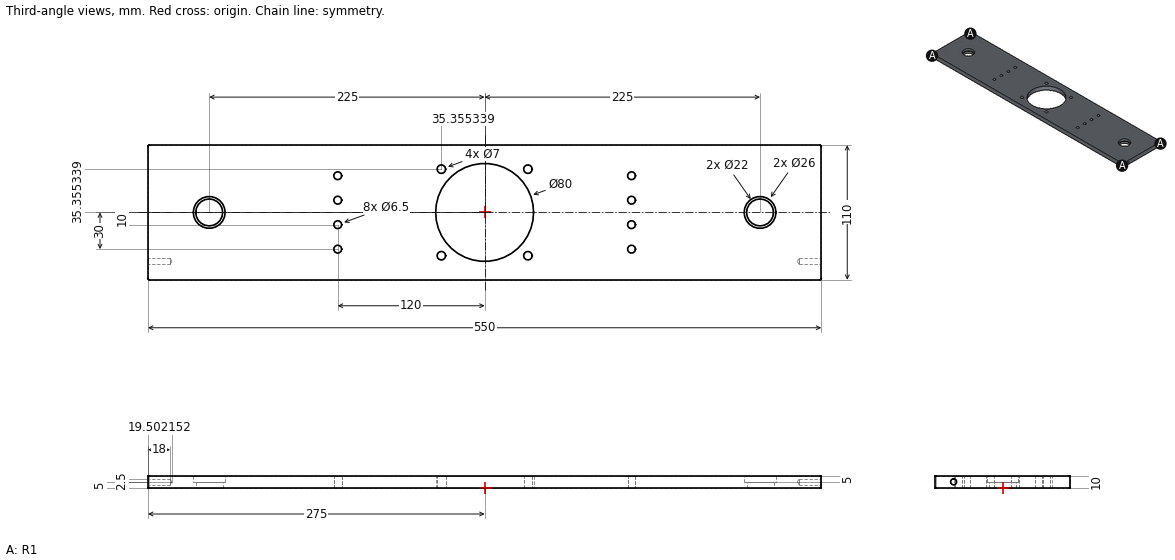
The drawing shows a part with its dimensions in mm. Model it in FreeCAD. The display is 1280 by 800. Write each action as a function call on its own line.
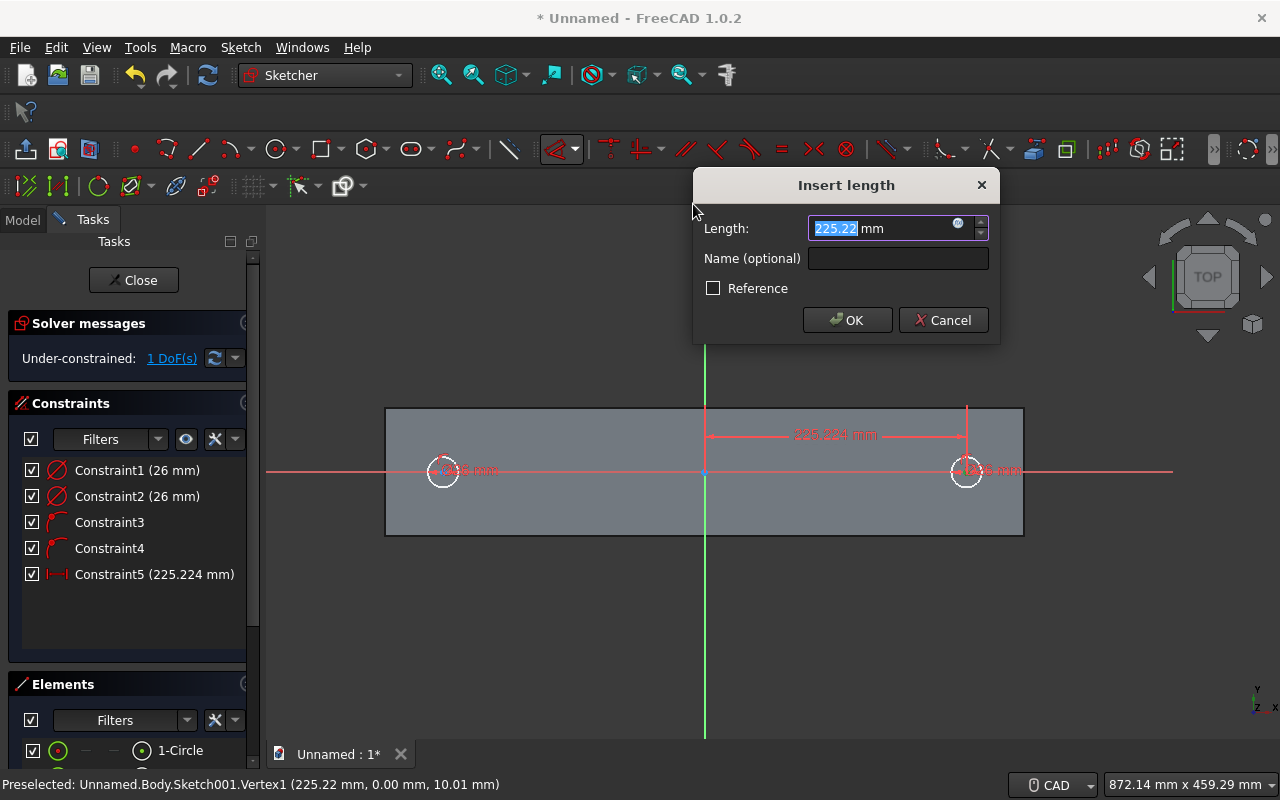
text(225)
key(Return)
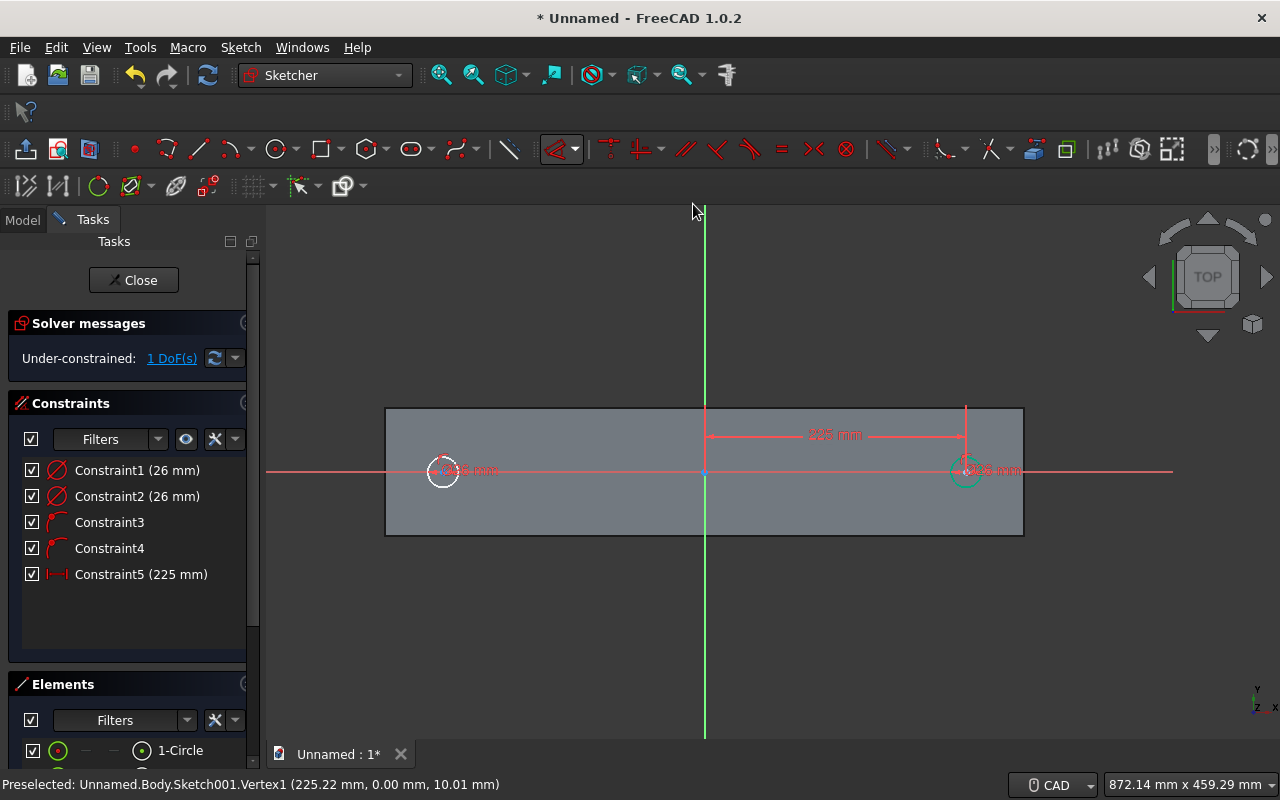
click(443, 472)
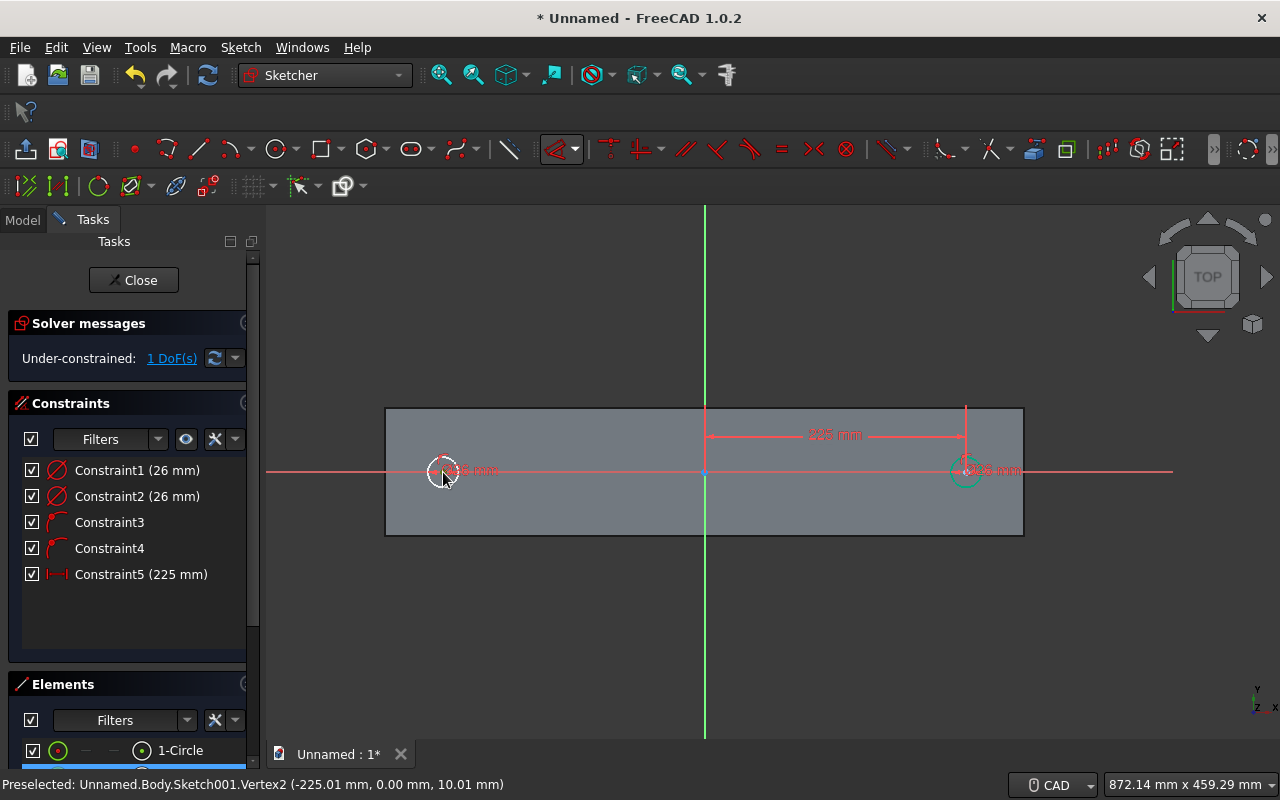
click(578, 150)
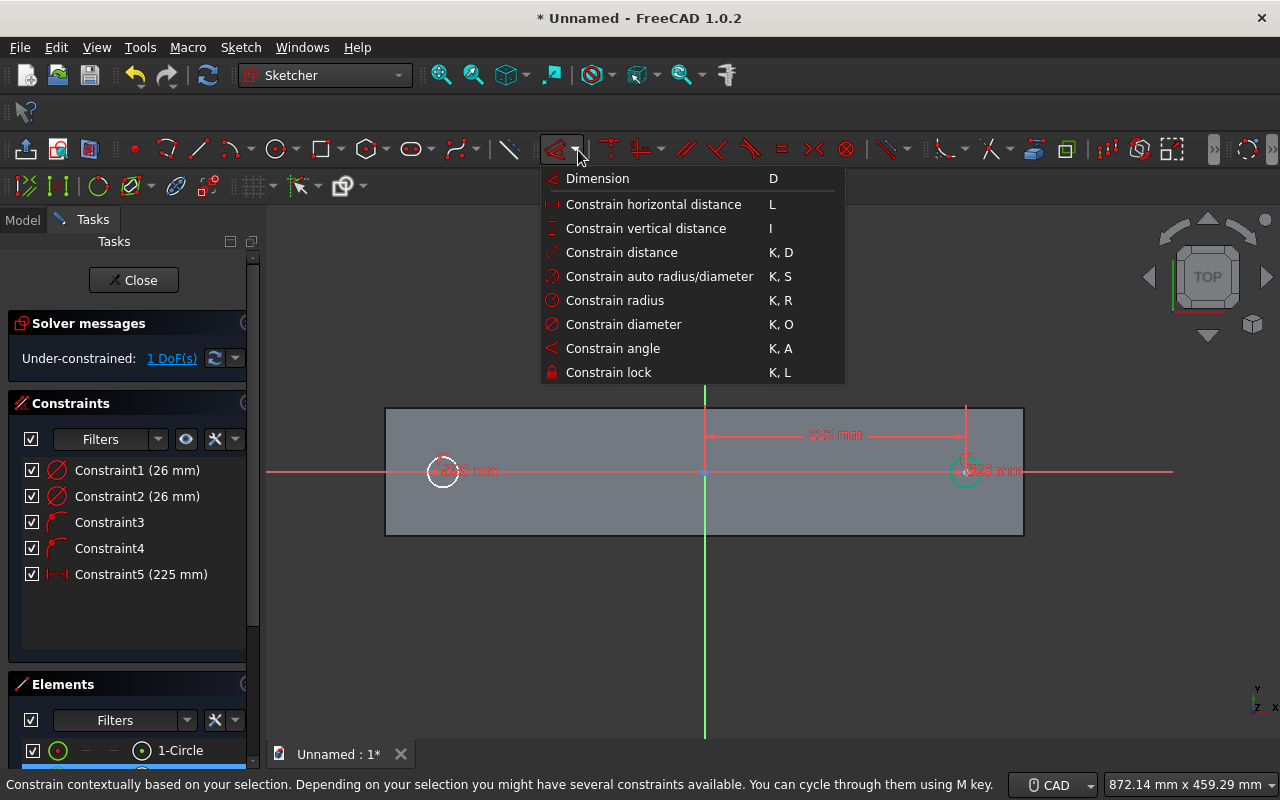
click(693, 204)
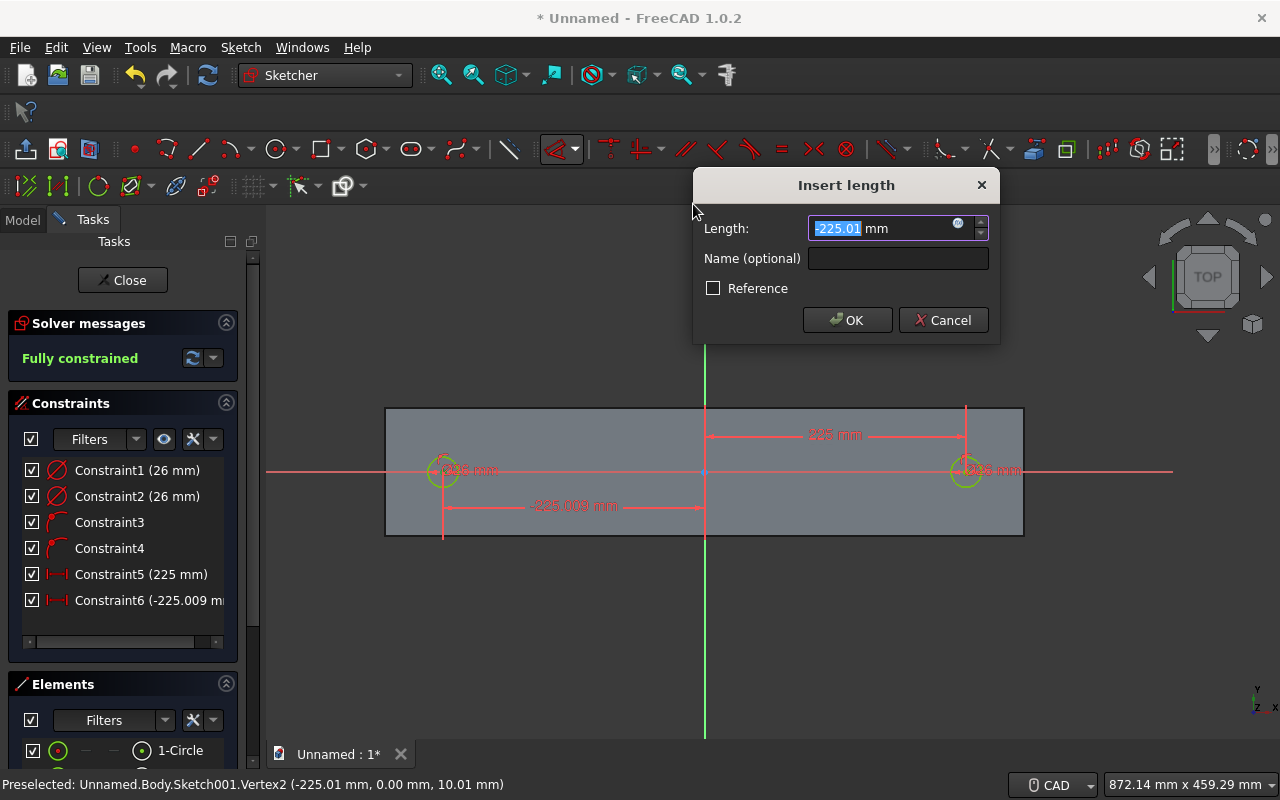
text(-225)
key(Return)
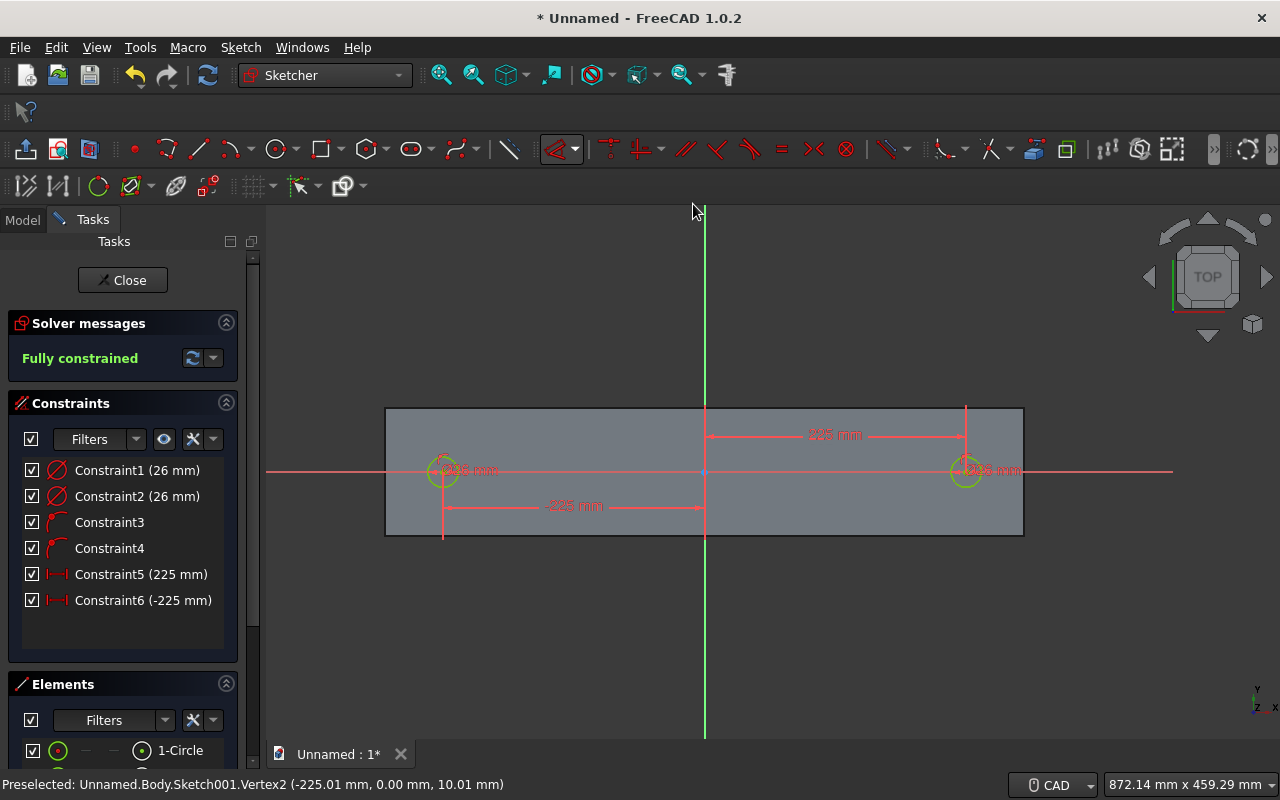
click(123, 280)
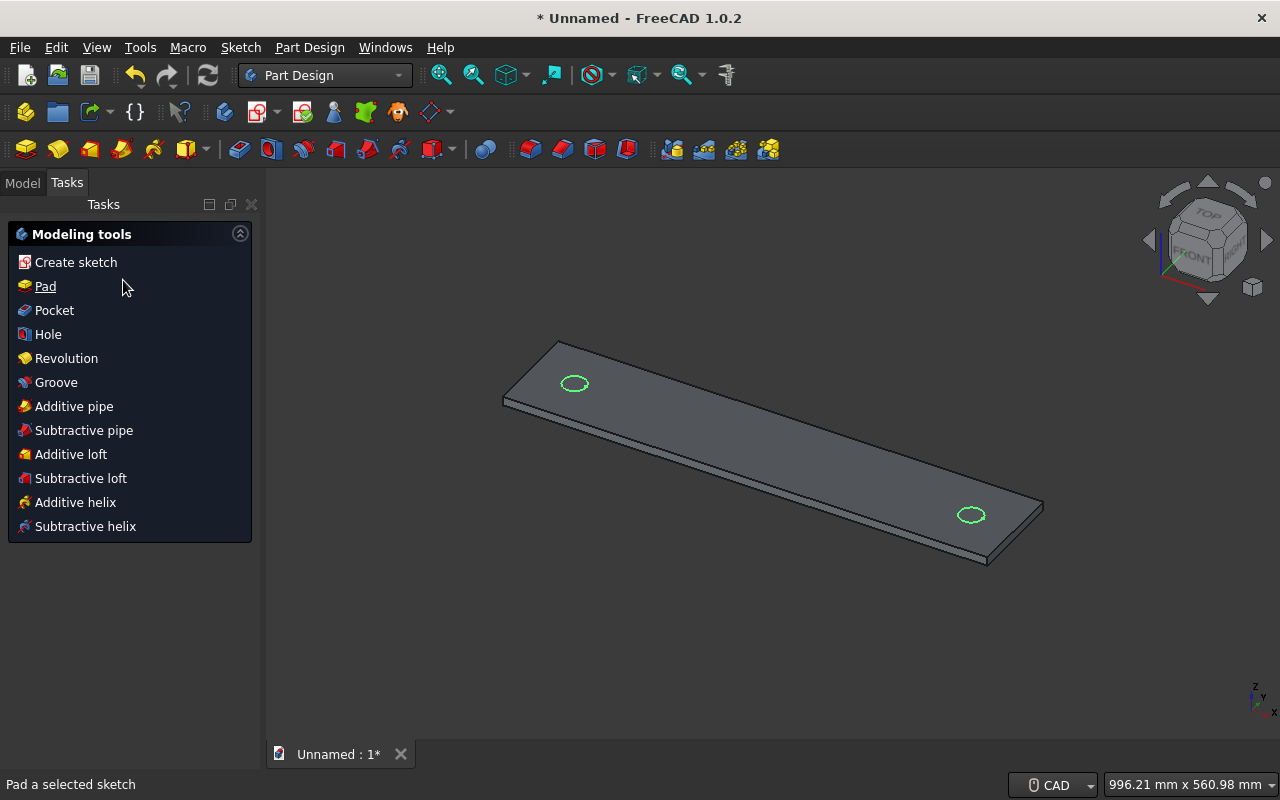
click(240, 150)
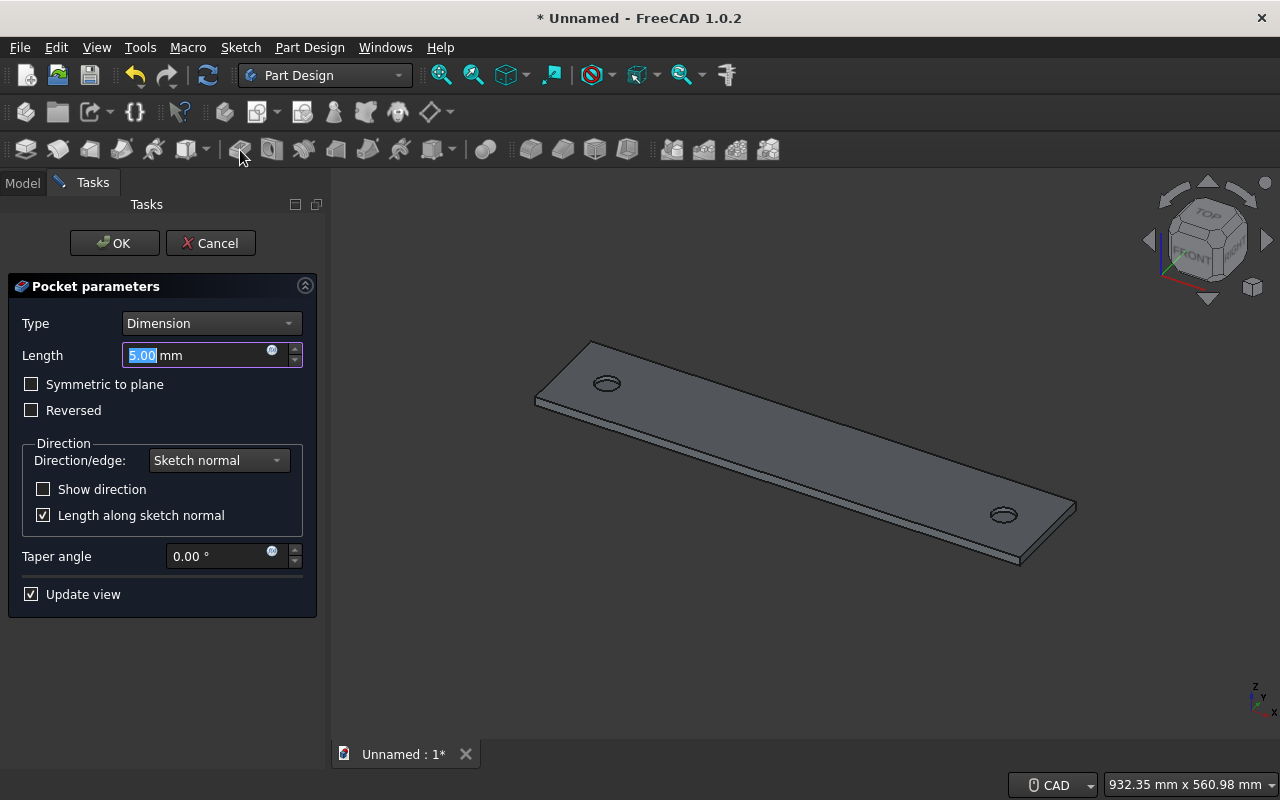
text(5)
key(Tab)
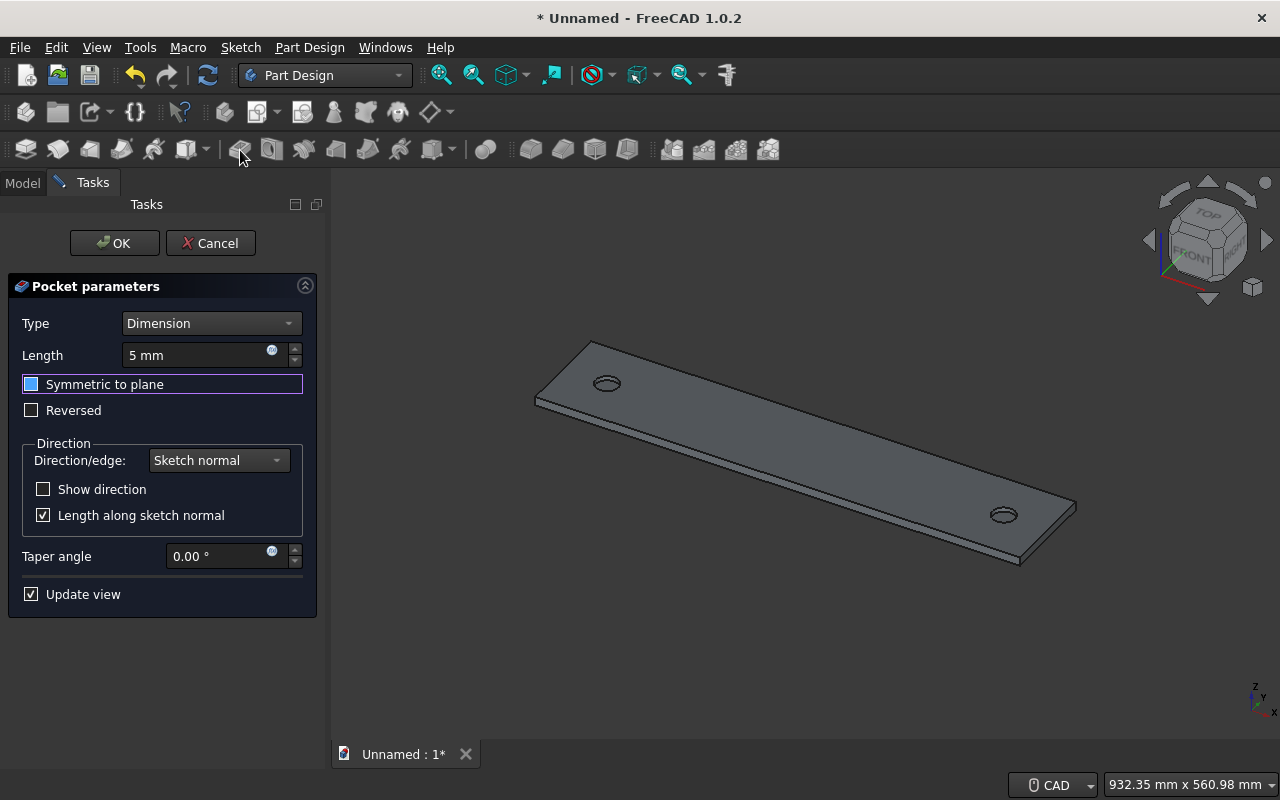
click(115, 243)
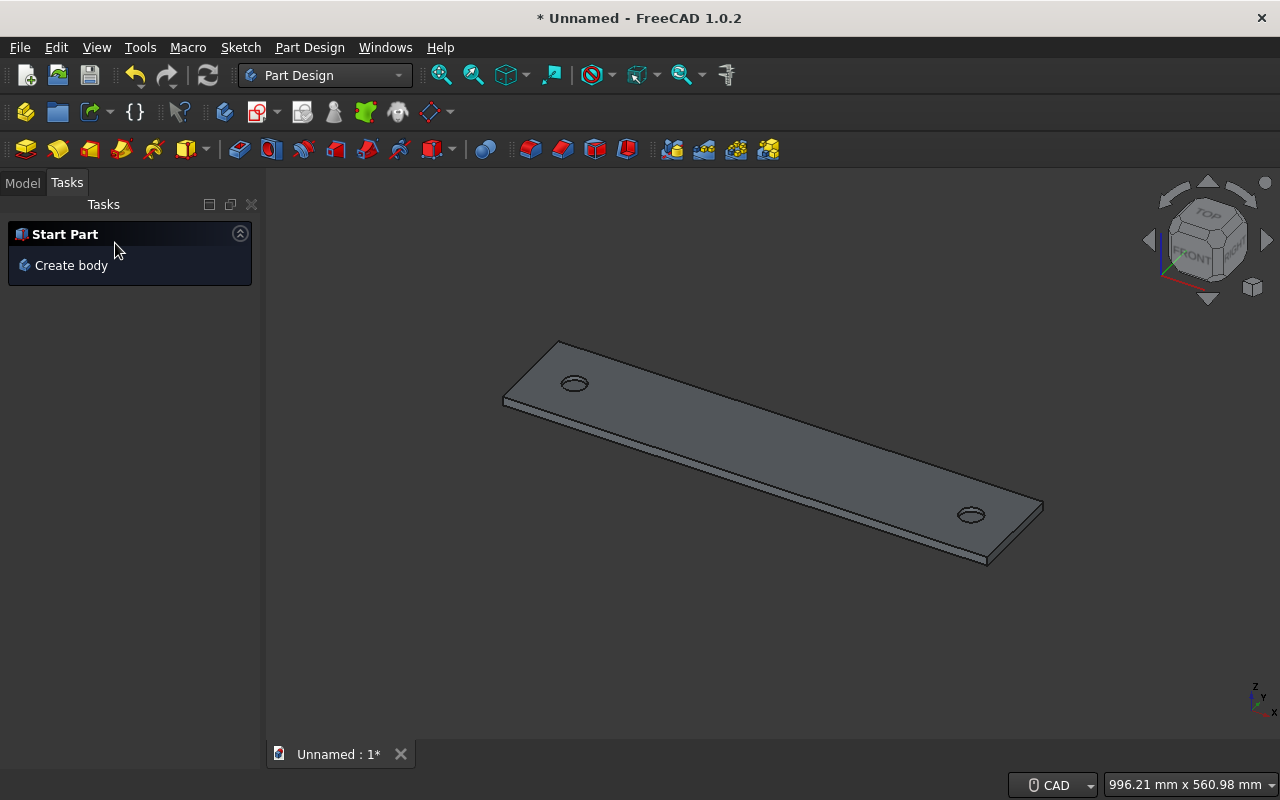
key(0)